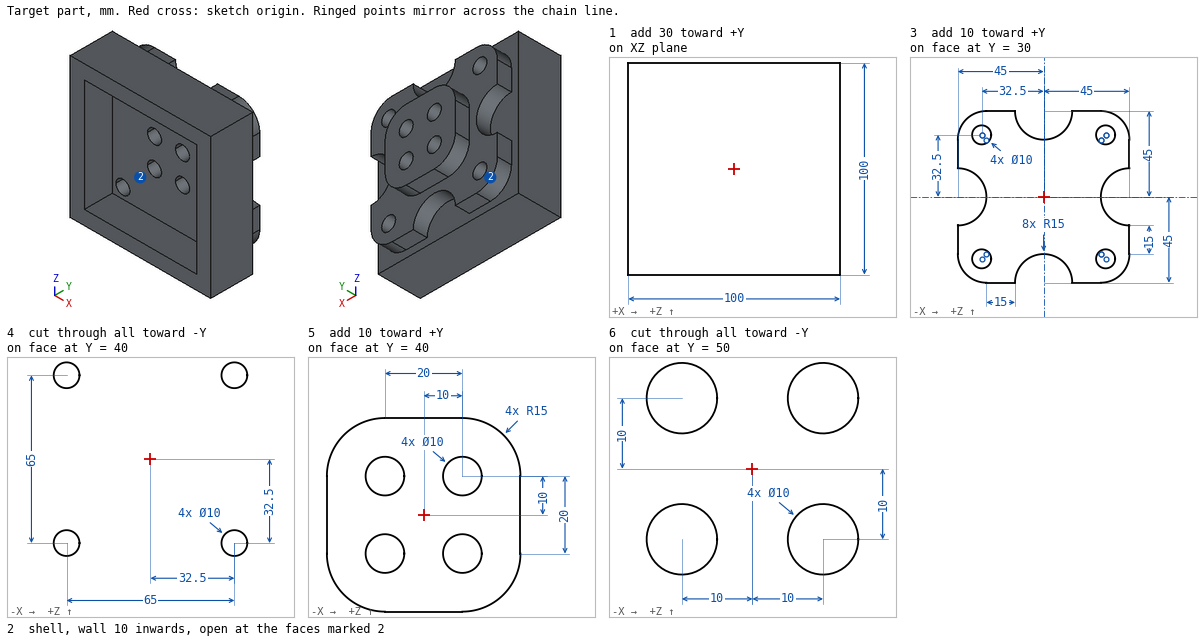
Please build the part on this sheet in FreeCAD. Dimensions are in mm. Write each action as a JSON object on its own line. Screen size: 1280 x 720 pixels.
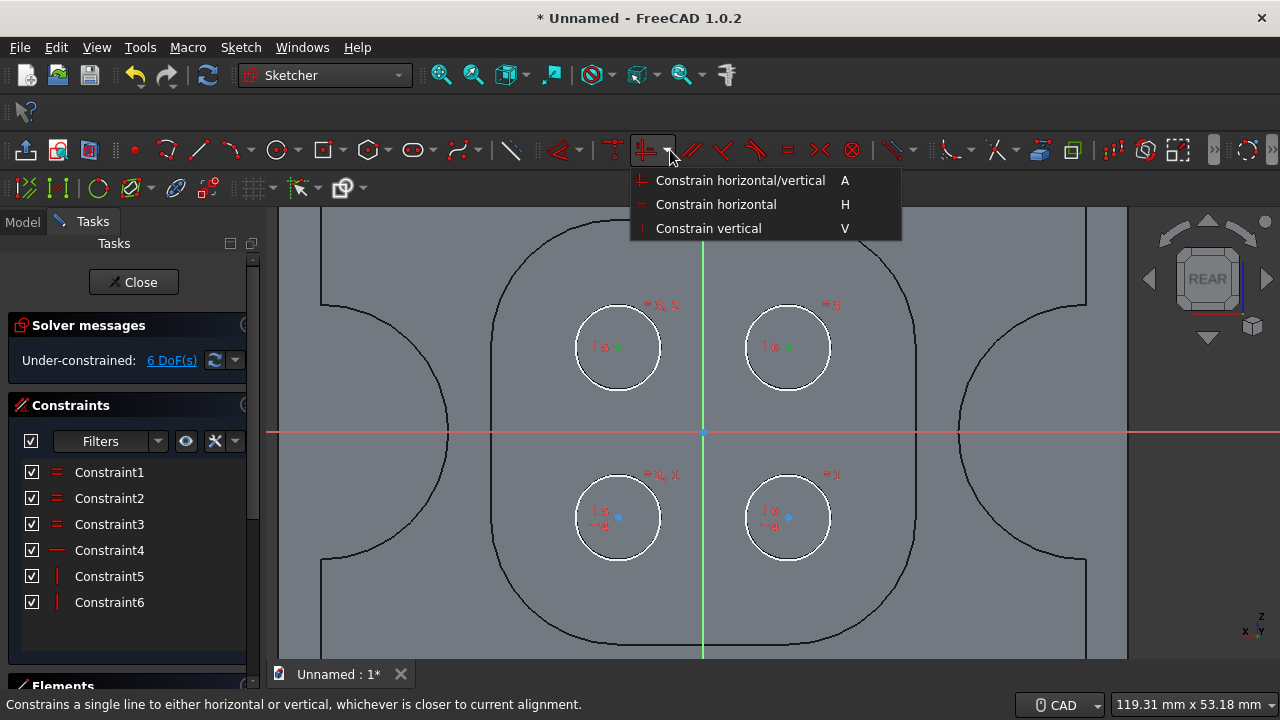
{"action": "left_click", "coordinate": [766, 204]}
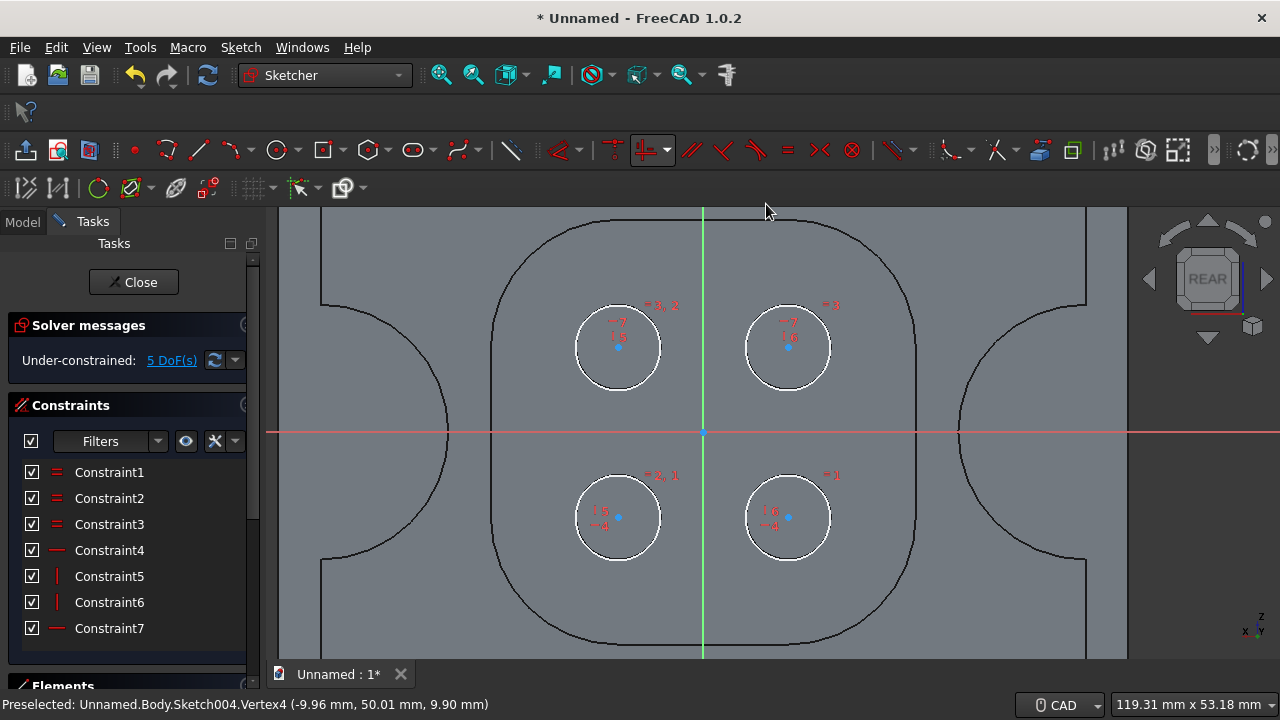
{"action": "left_click", "coordinate": [558, 150]}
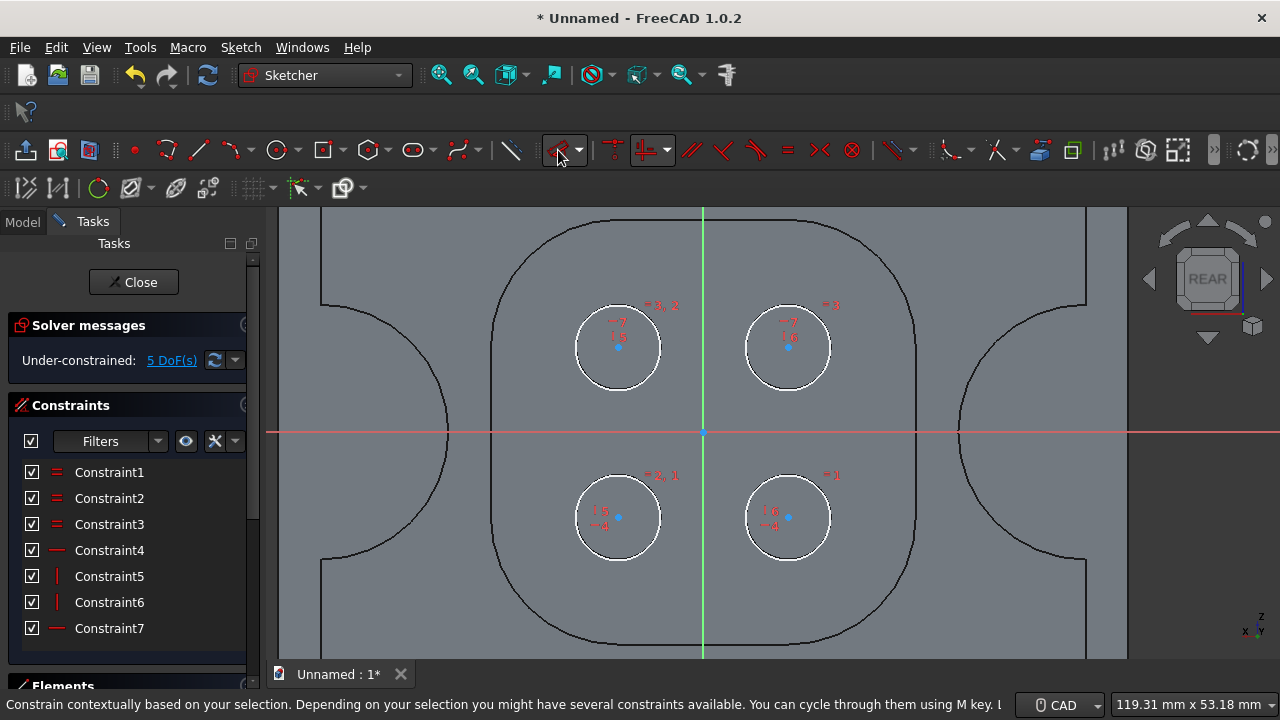
{"action": "left_click", "coordinate": [818, 488]}
{"action": "left_click", "coordinate": [841, 465]}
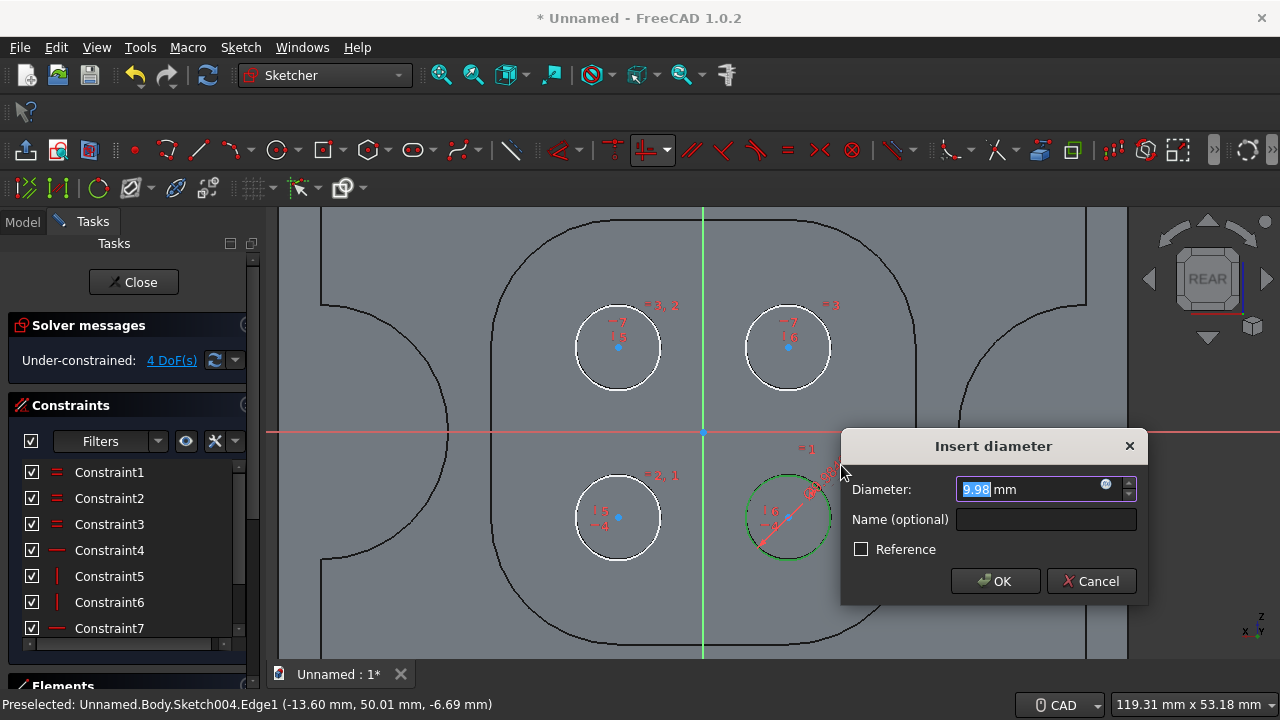
{"action": "type", "text": "10"}
{"action": "key", "text": "Return"}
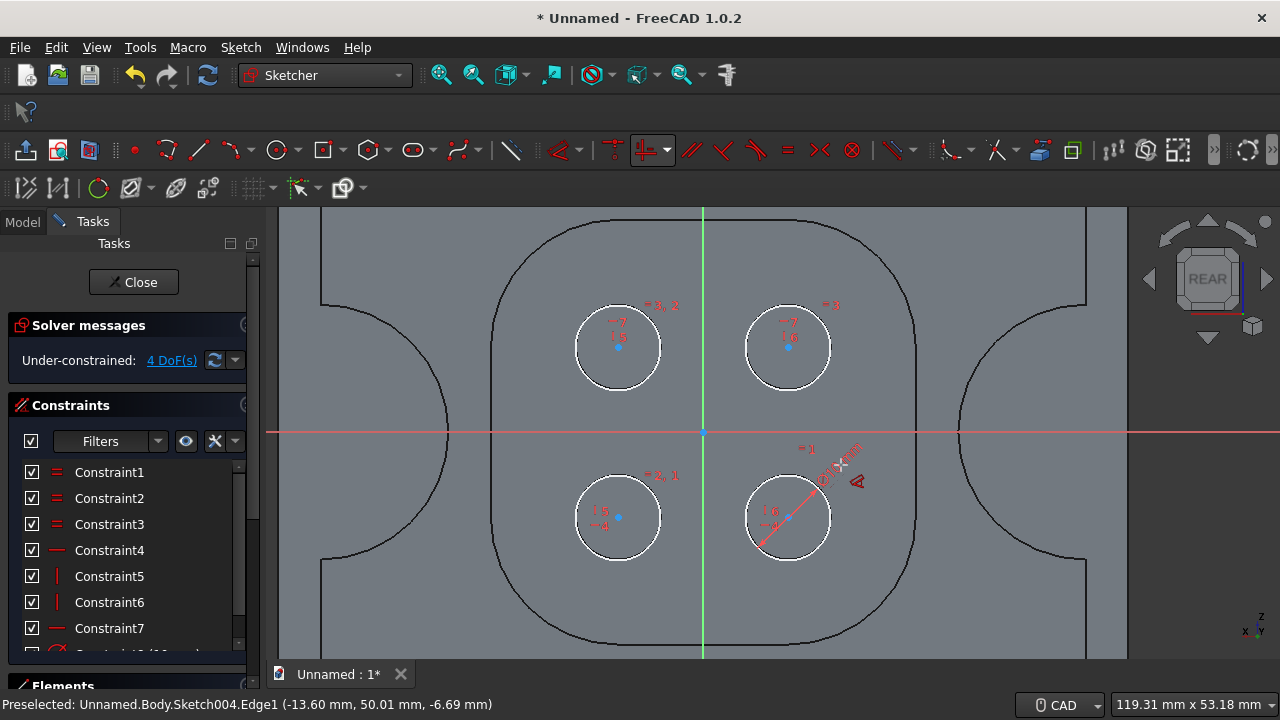
{"action": "left_click", "coordinate": [788, 518]}
{"action": "left_click", "coordinate": [726, 552]}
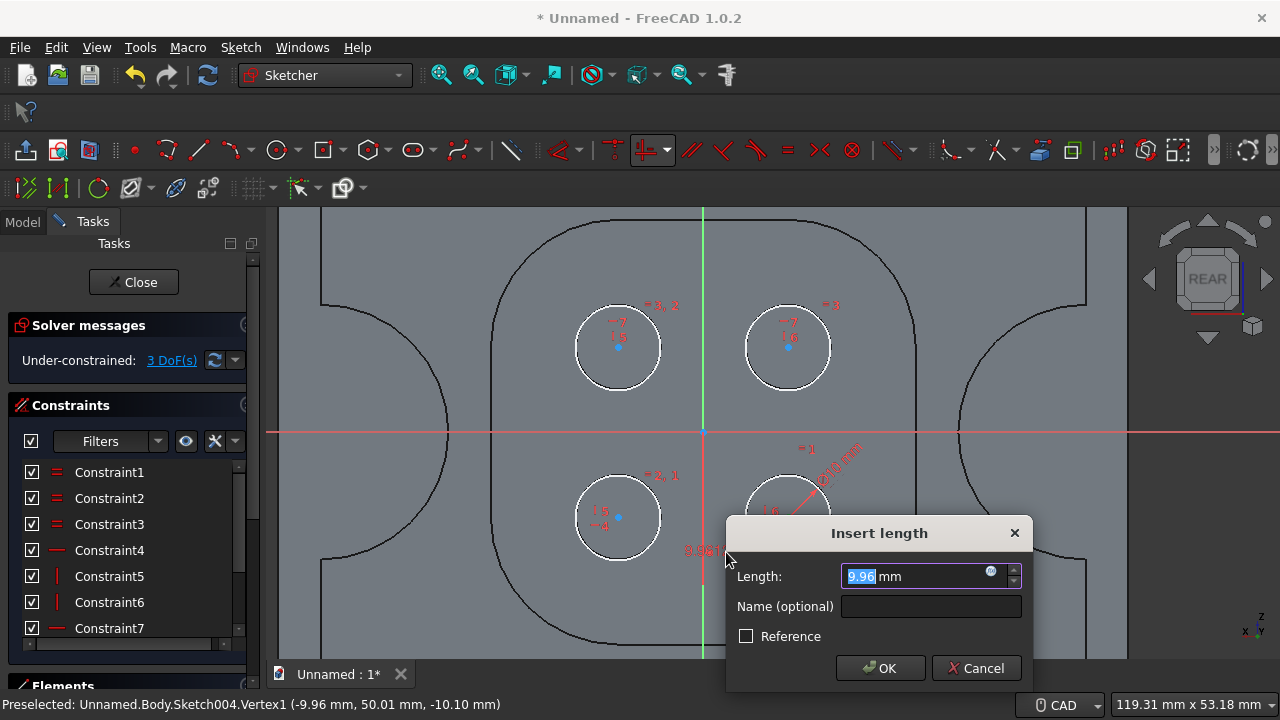
{"action": "type", "text": "10"}
{"action": "key", "text": "Return"}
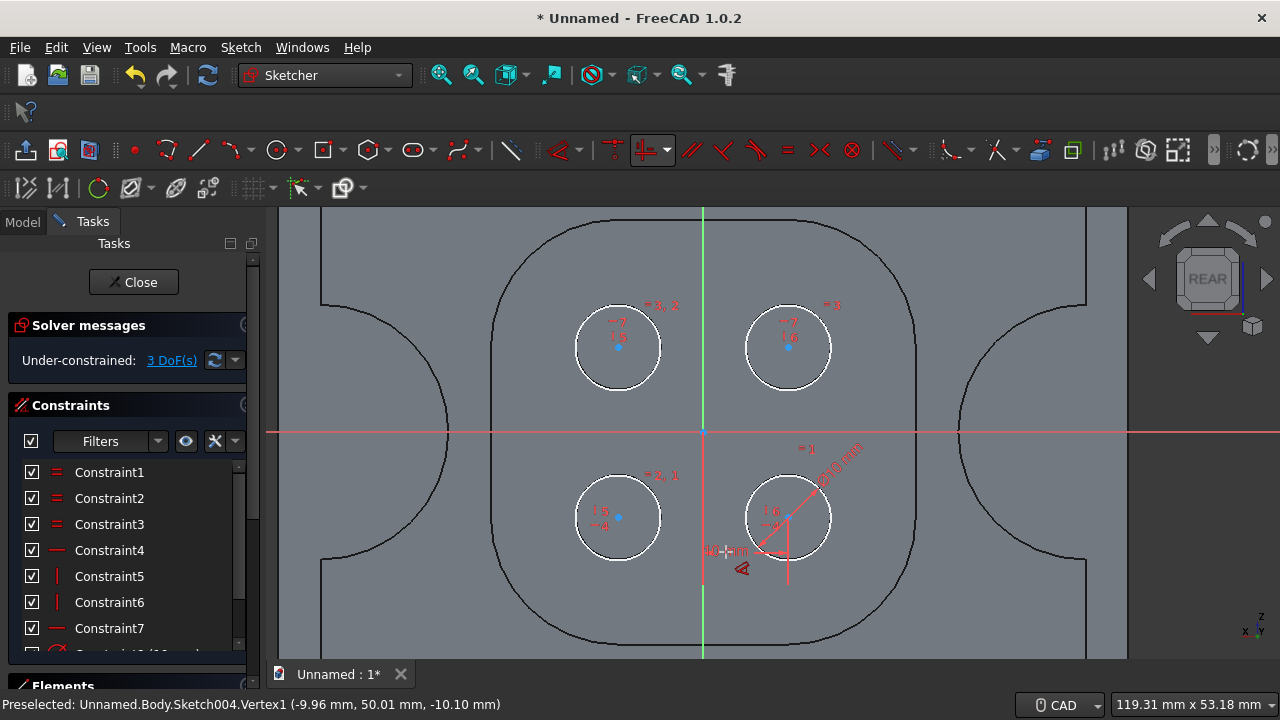
{"action": "left_click", "coordinate": [788, 518]}
{"action": "left_click", "coordinate": [669, 475]}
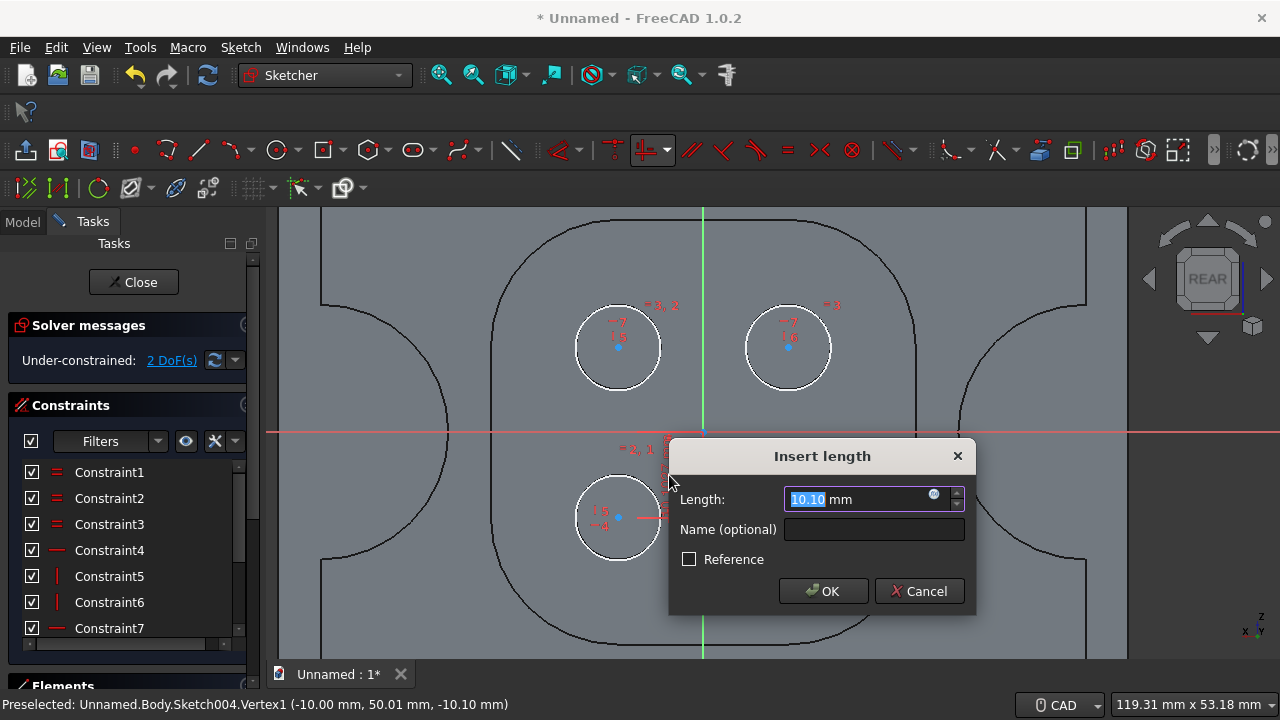
{"action": "type", "text": "10"}
{"action": "key", "text": "Return"}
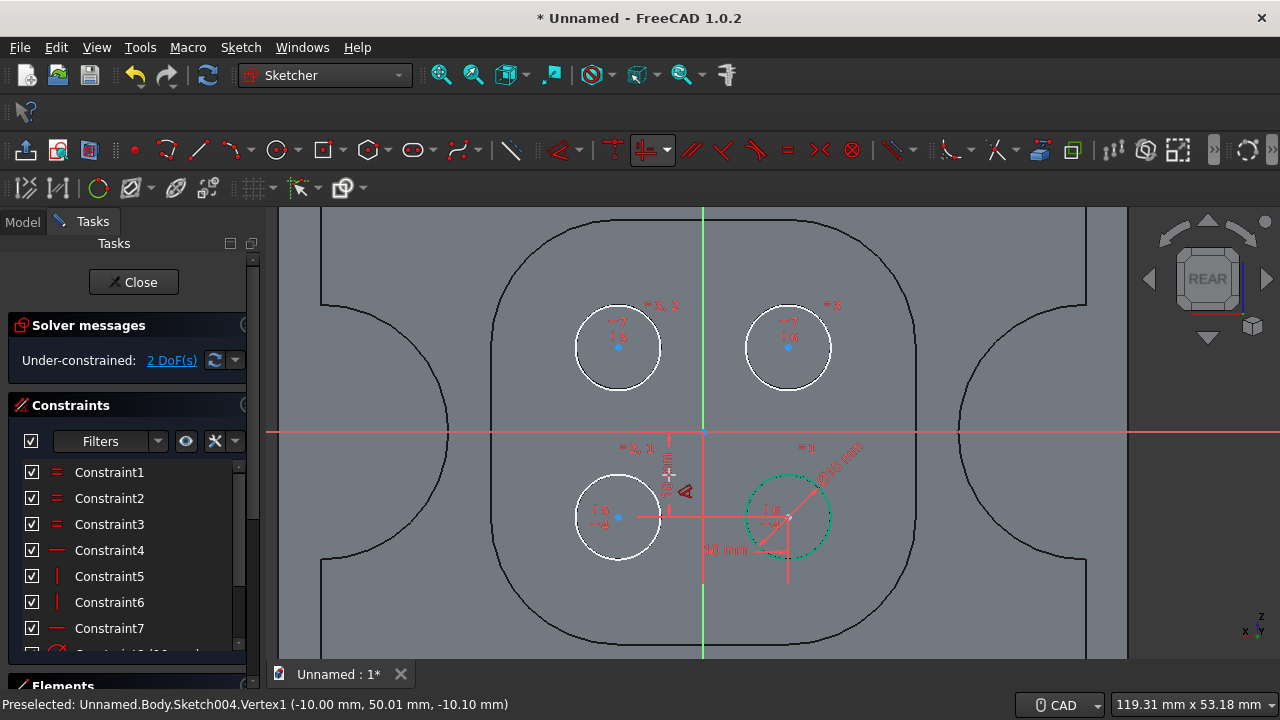
{"action": "left_click", "coordinate": [618, 517]}
{"action": "left_click", "coordinate": [661, 398]}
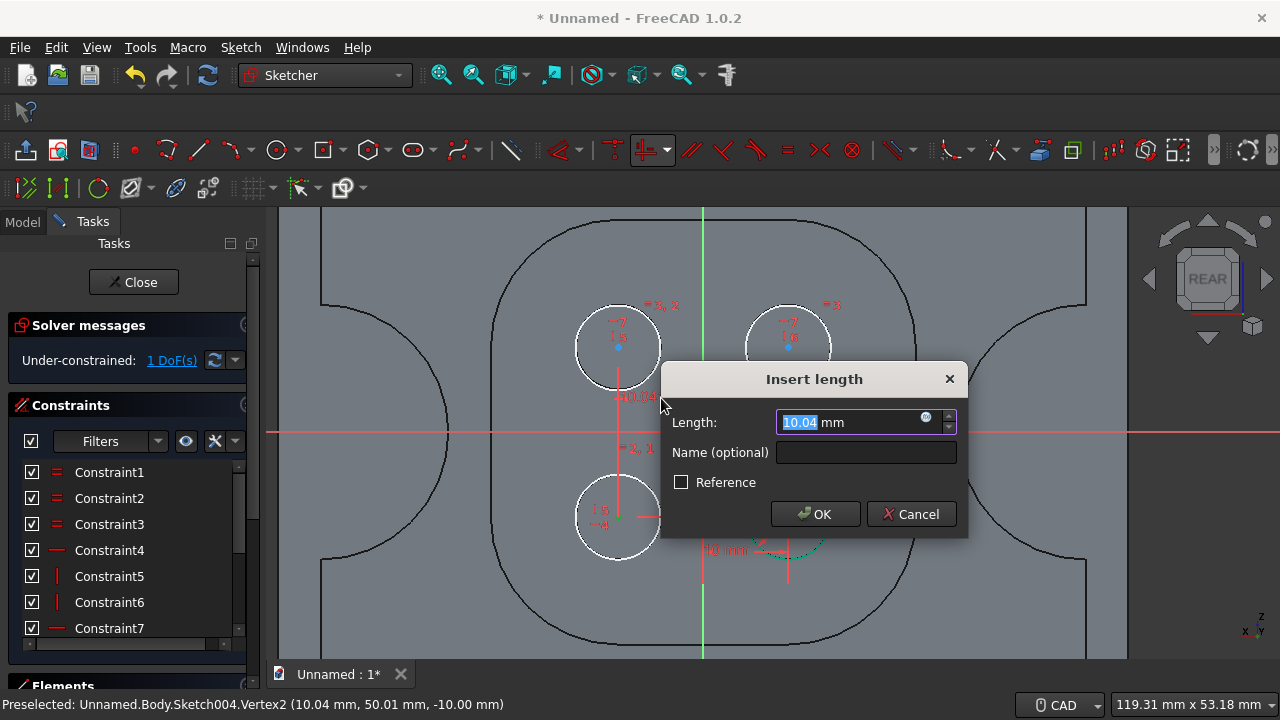
{"action": "type", "text": "10"}
{"action": "key", "text": "Return"}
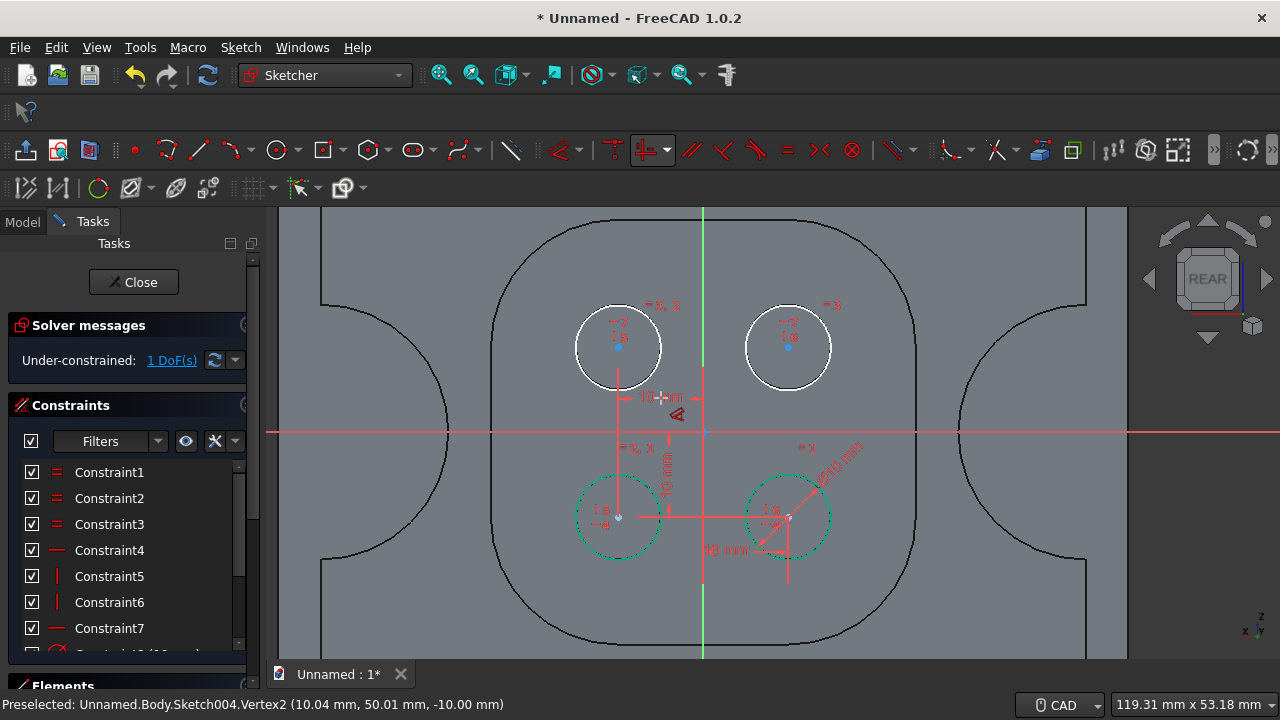
{"action": "left_click", "coordinate": [618, 348]}
{"action": "left_click", "coordinate": [584, 409]}